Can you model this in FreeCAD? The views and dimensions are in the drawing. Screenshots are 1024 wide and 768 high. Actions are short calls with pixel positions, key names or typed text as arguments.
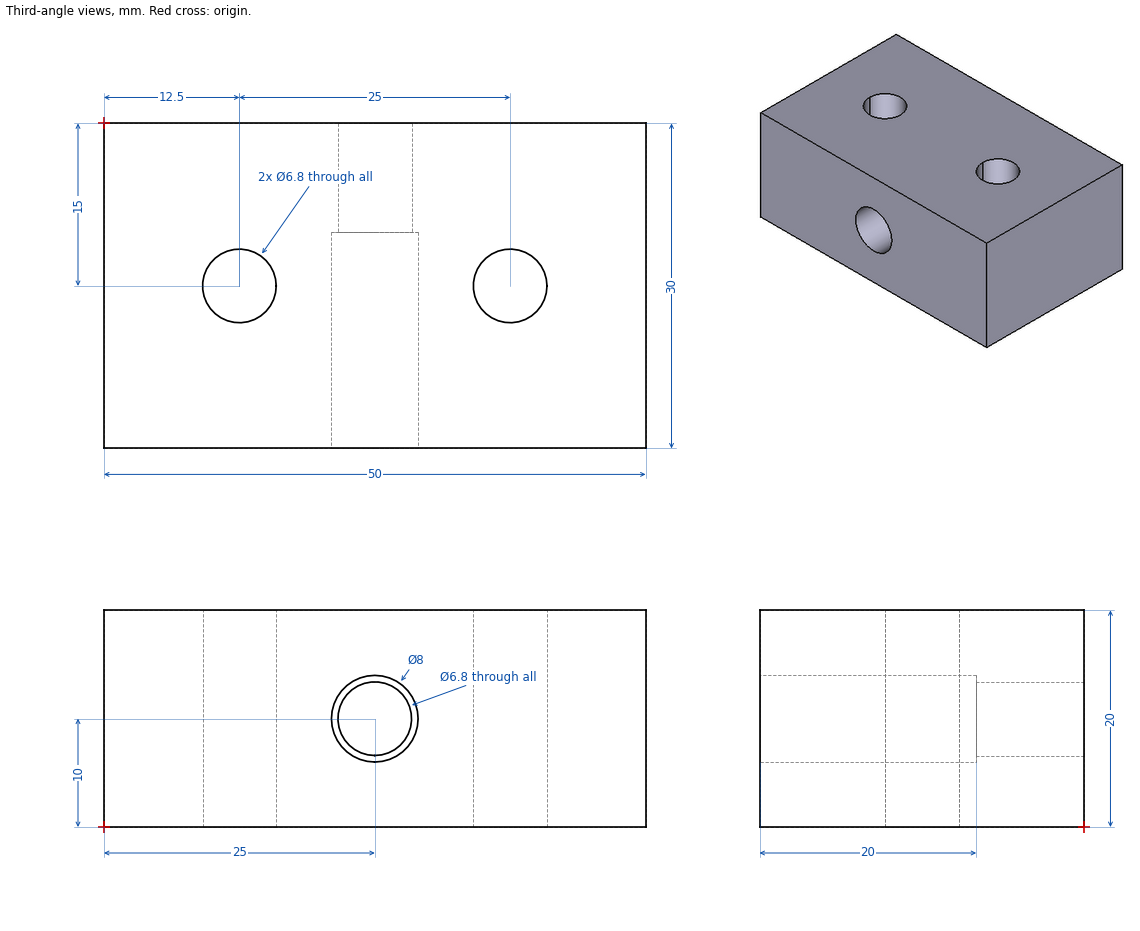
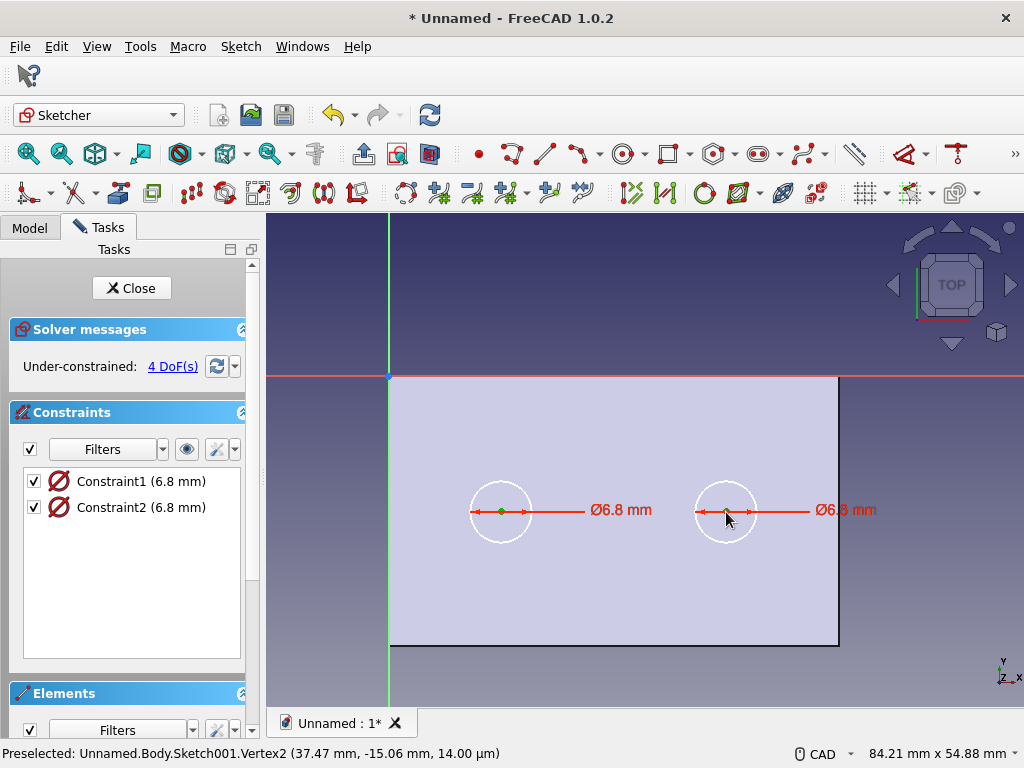
key(h)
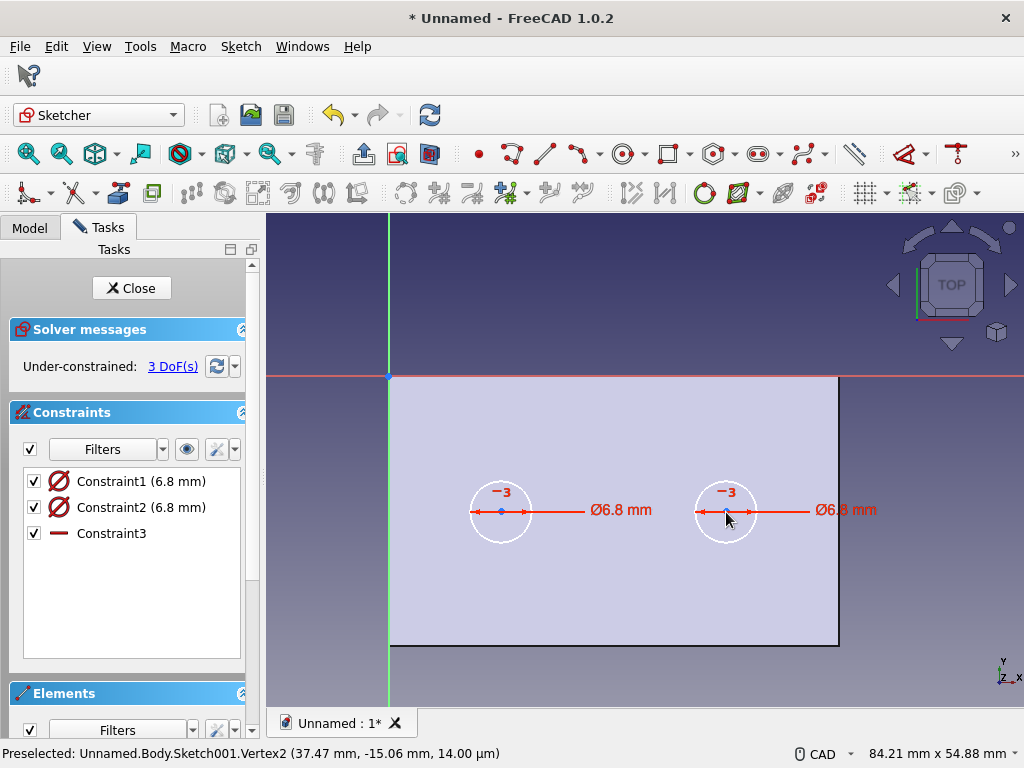
click(904, 154)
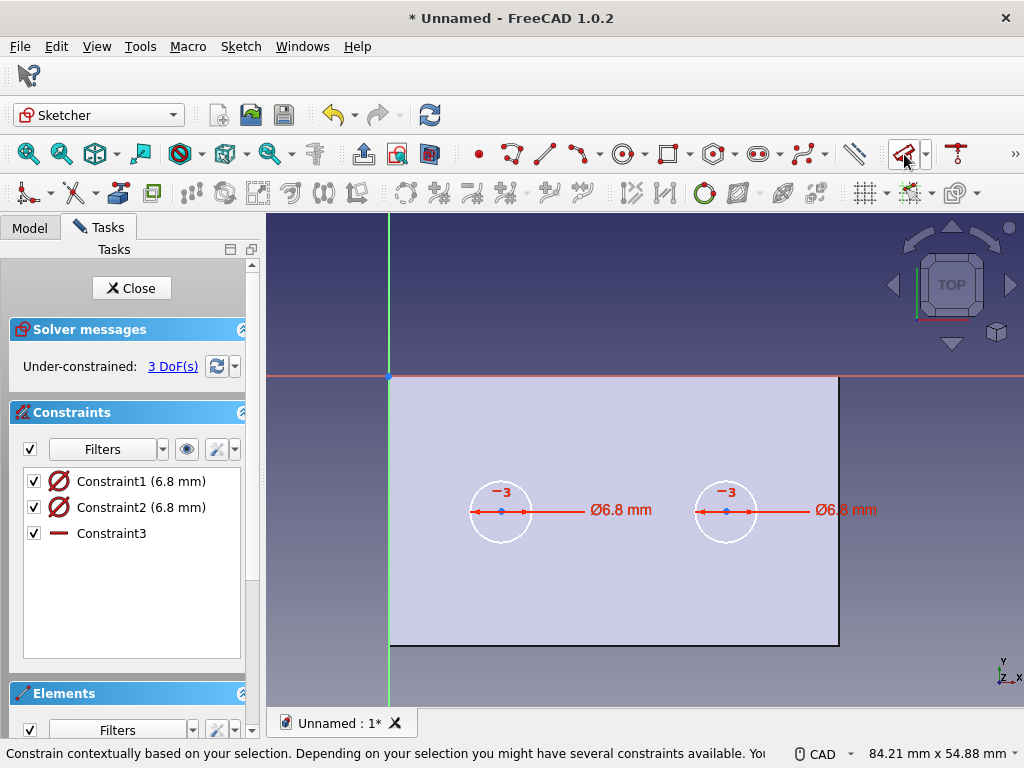
click(501, 512)
click(355, 444)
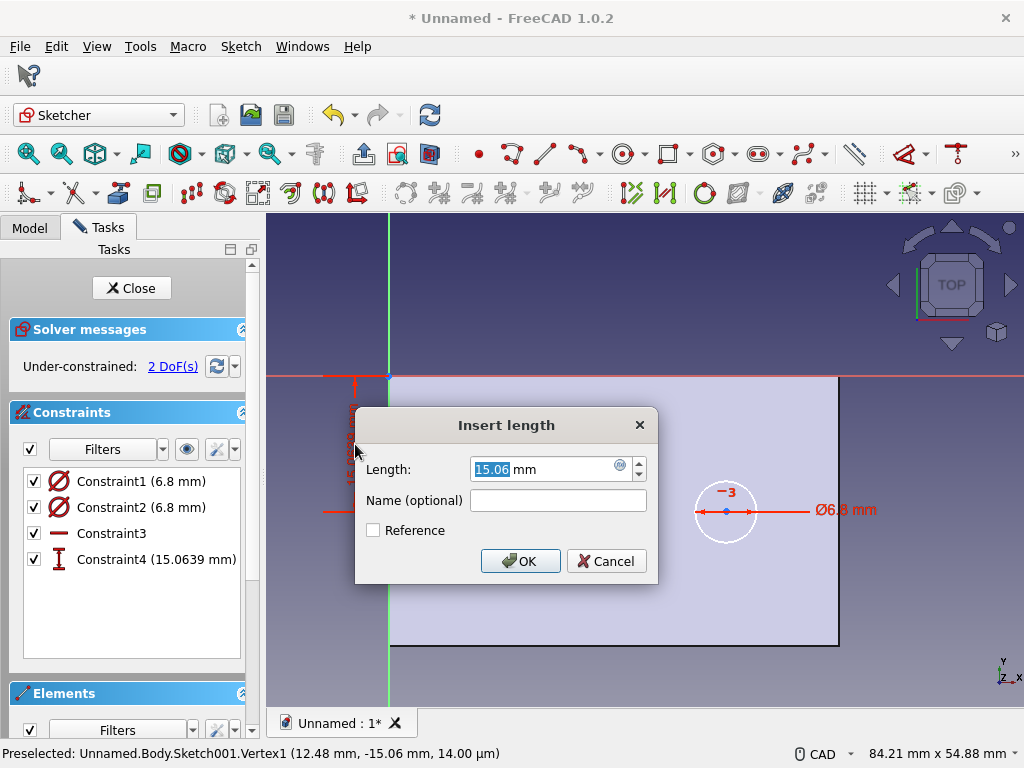
text(15)
key(Return)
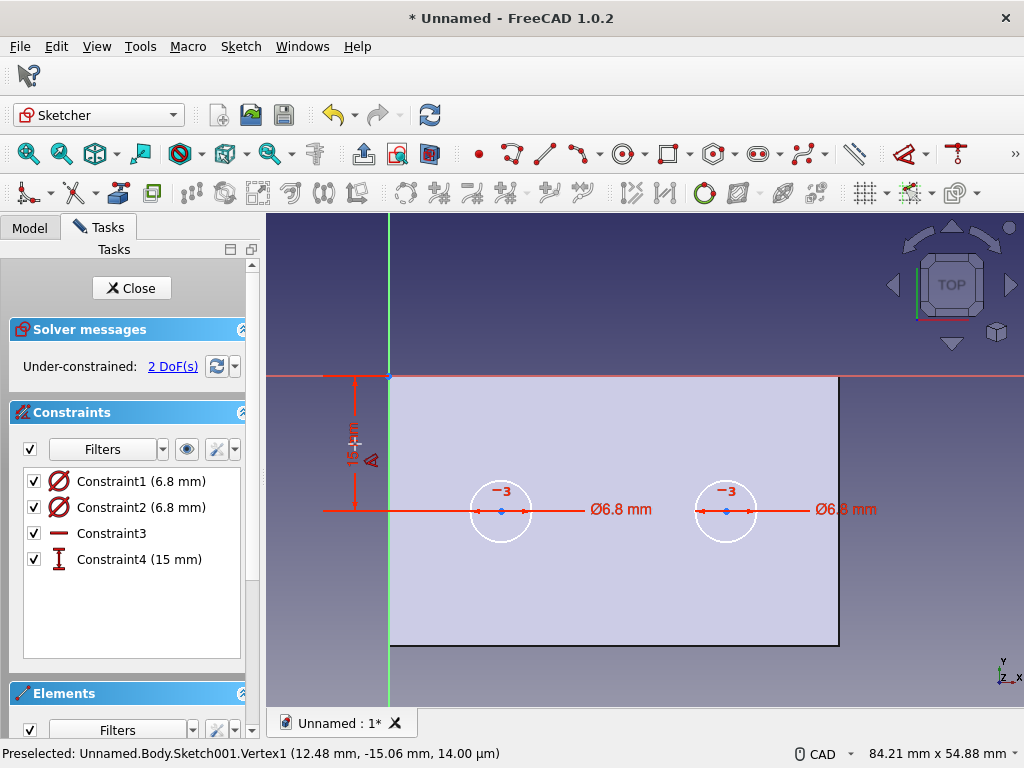
click(501, 511)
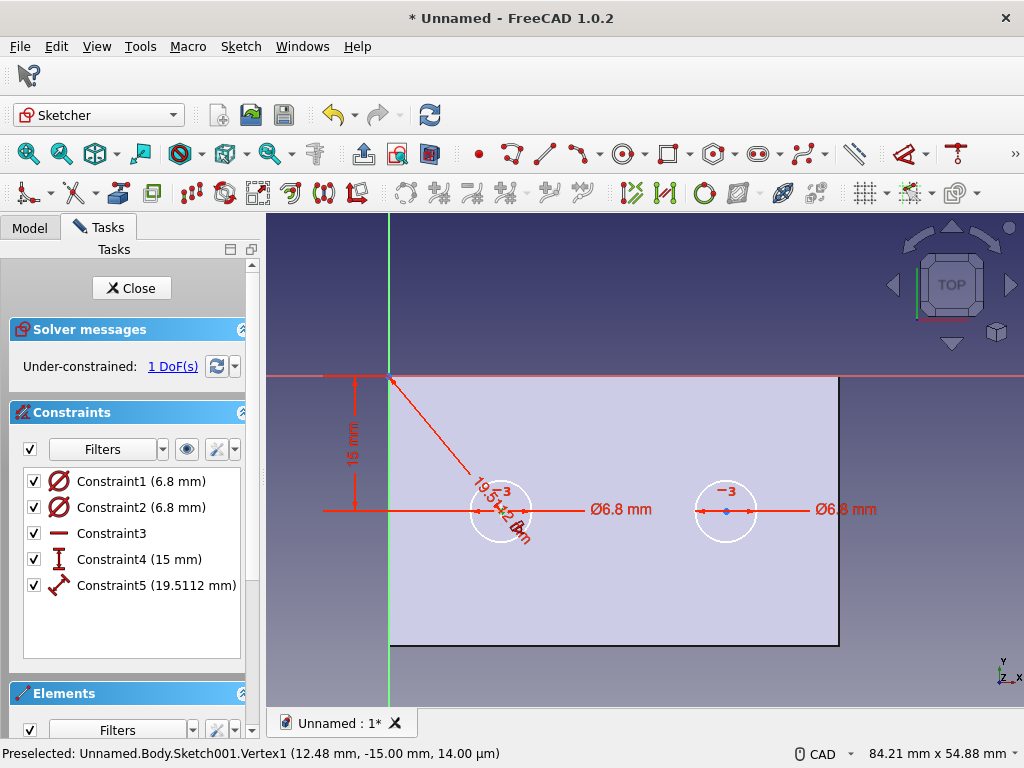
click(726, 511)
click(613, 545)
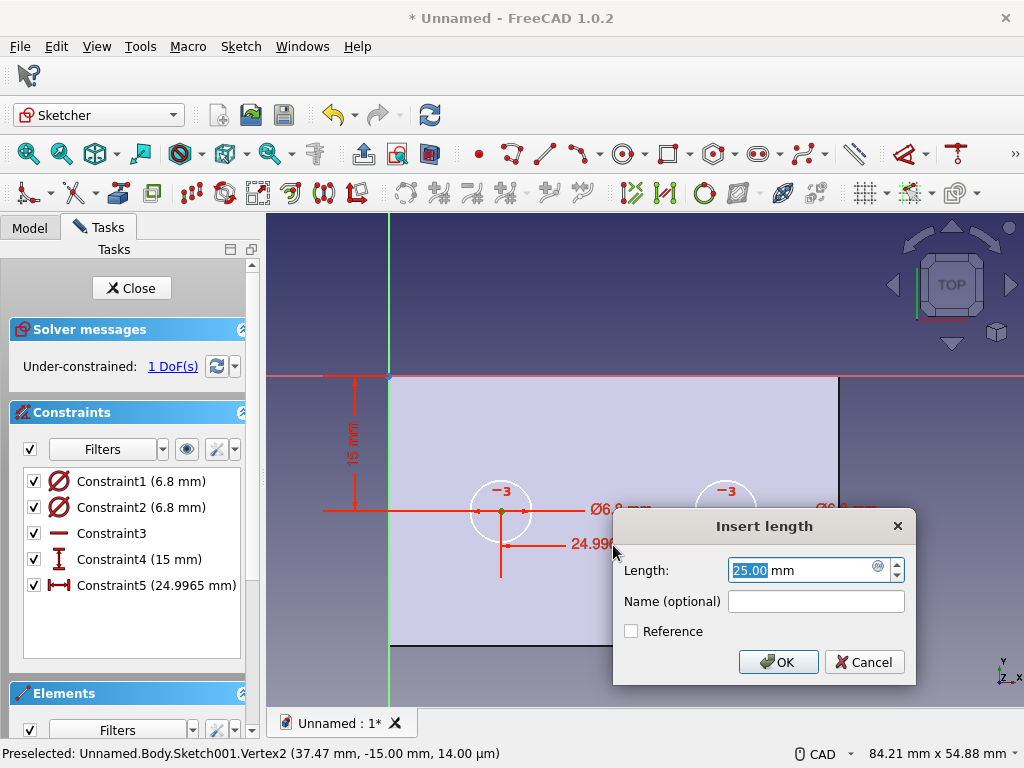
text(25)
key(Return)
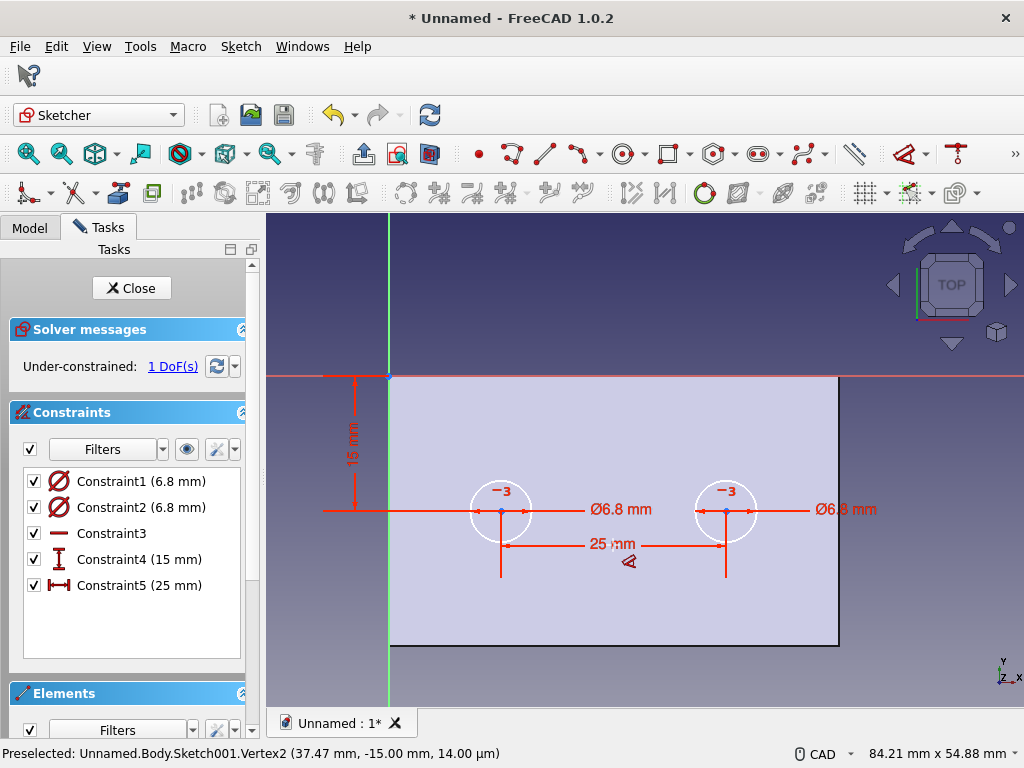
click(501, 511)
click(445, 342)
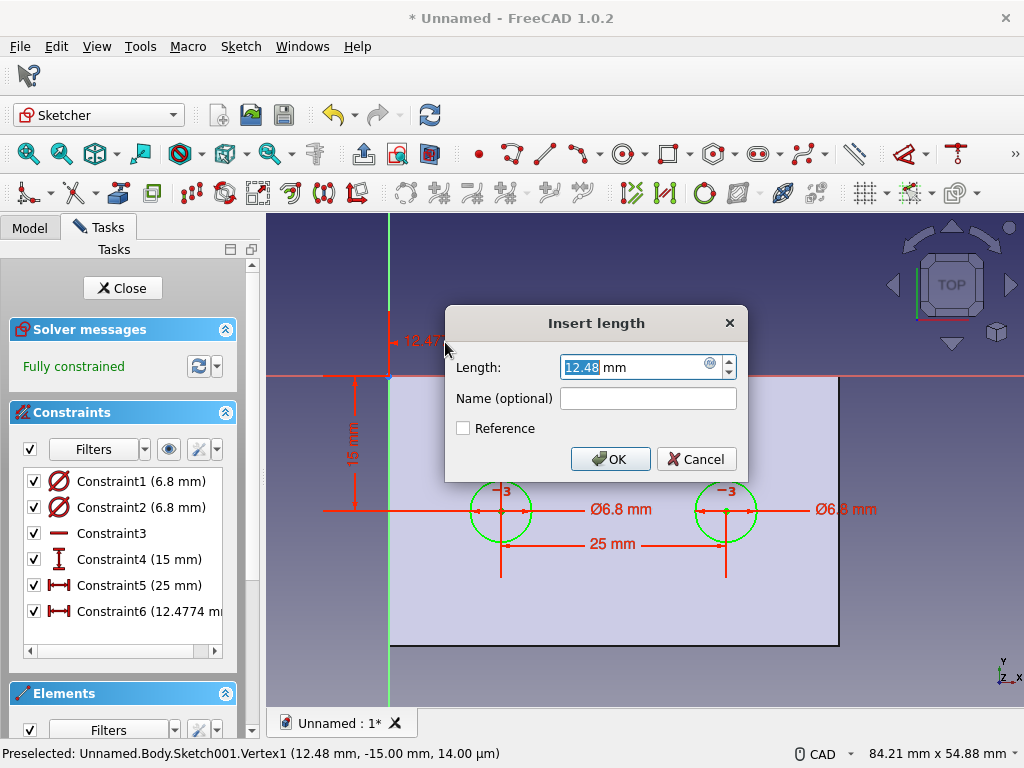
text(12.5)
key(Return)
key(Escape)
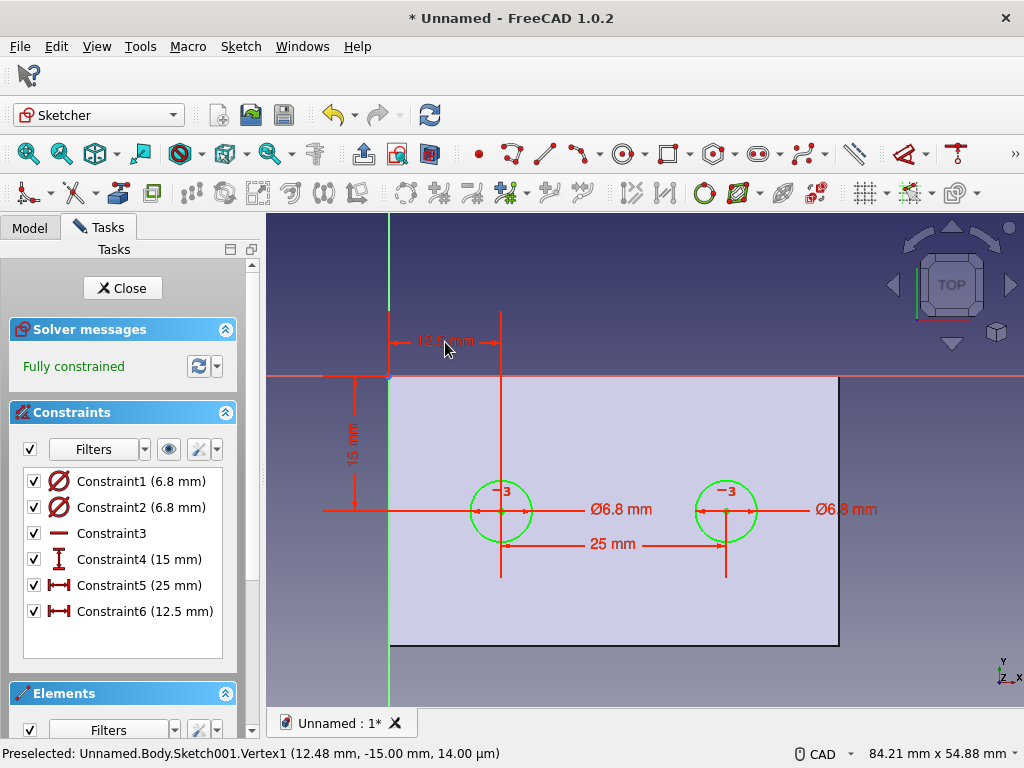
click(123, 288)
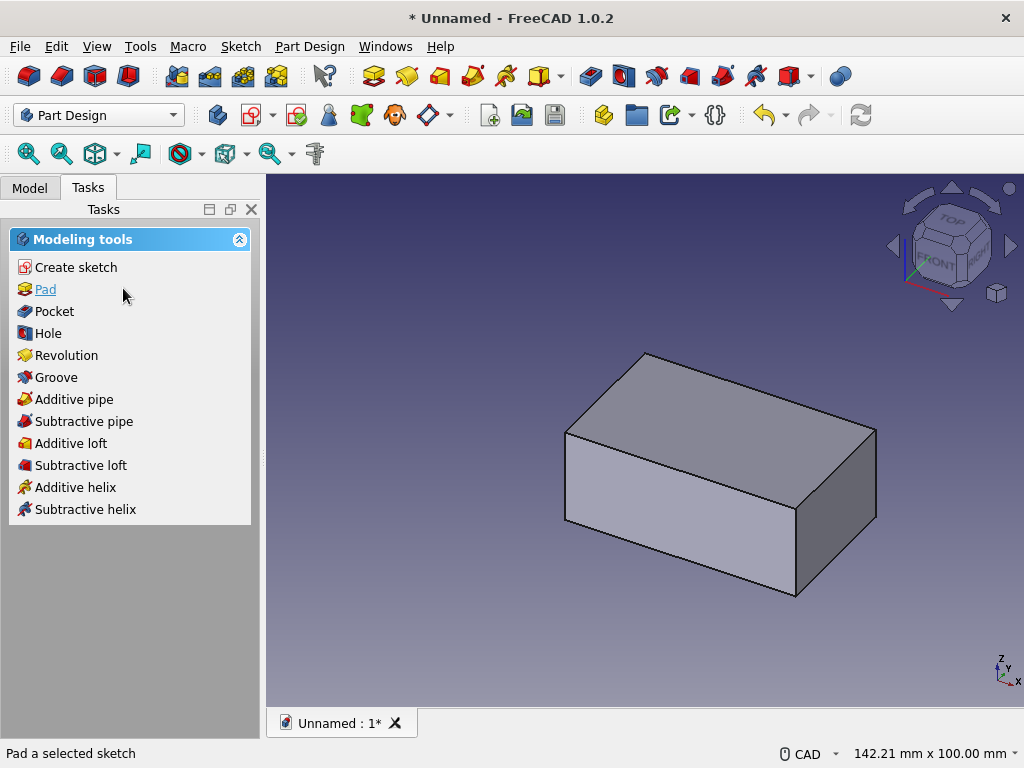
click(624, 76)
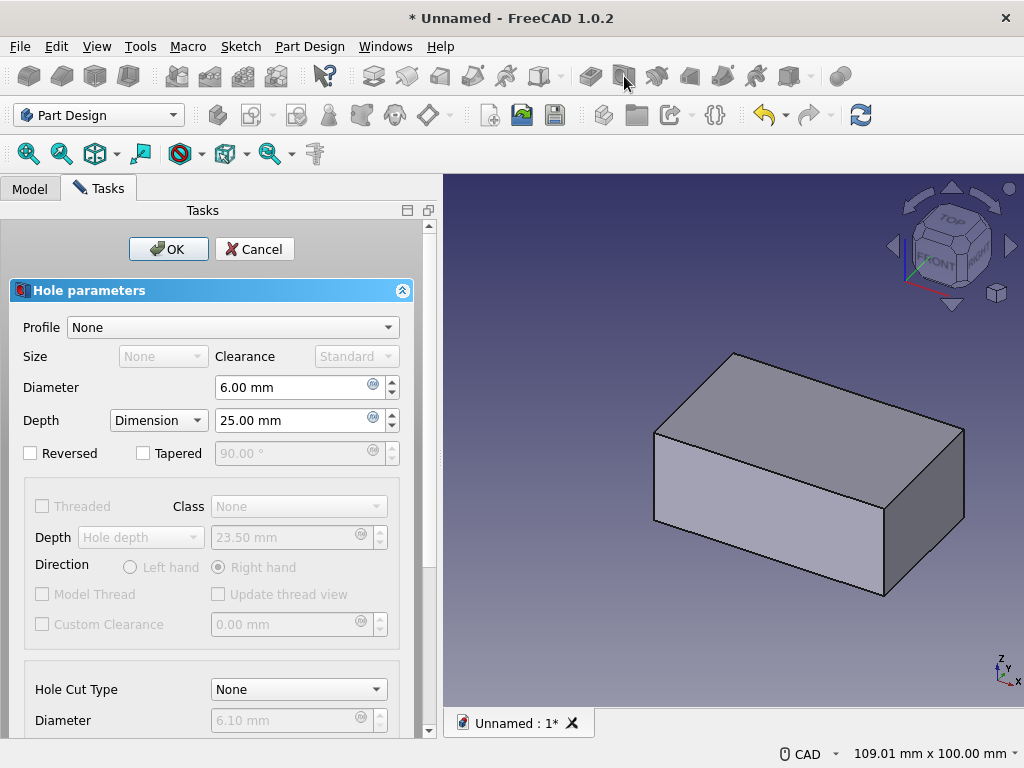
triple_click(300, 388)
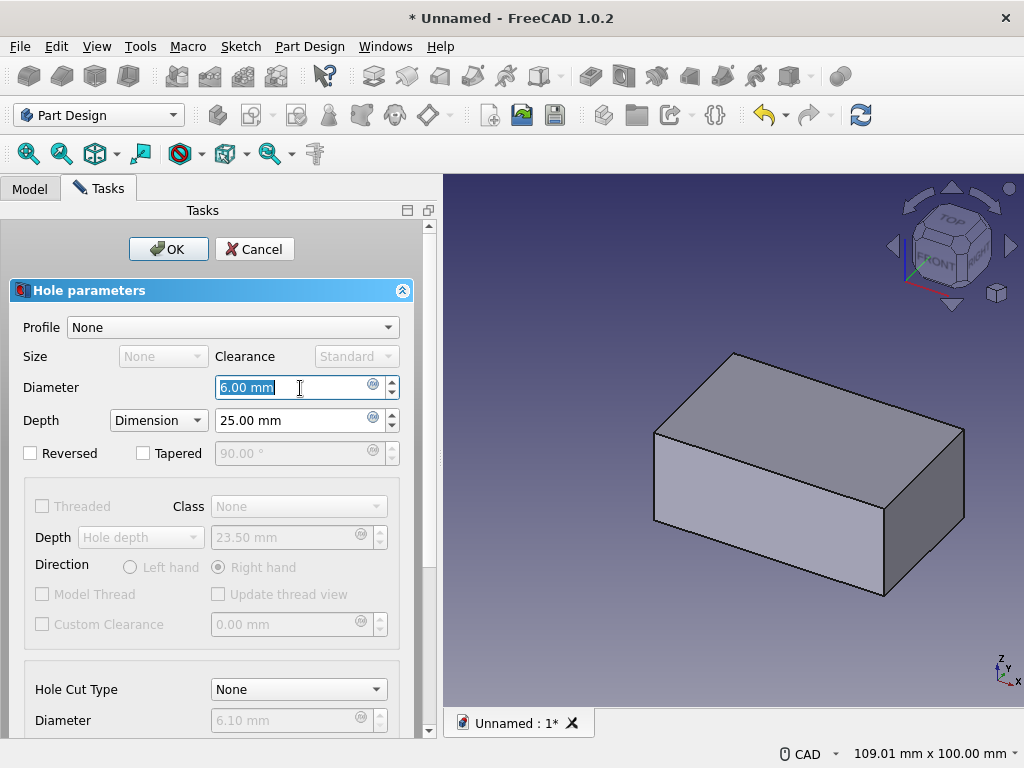
text(6.8)
key(Tab)